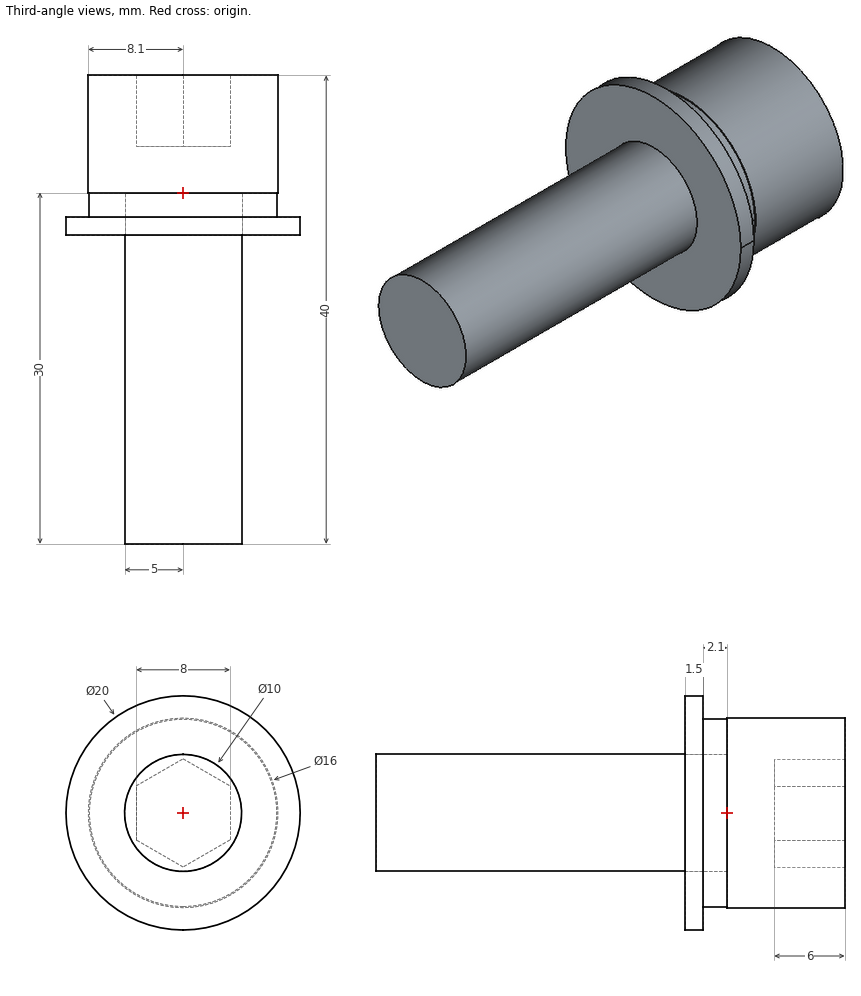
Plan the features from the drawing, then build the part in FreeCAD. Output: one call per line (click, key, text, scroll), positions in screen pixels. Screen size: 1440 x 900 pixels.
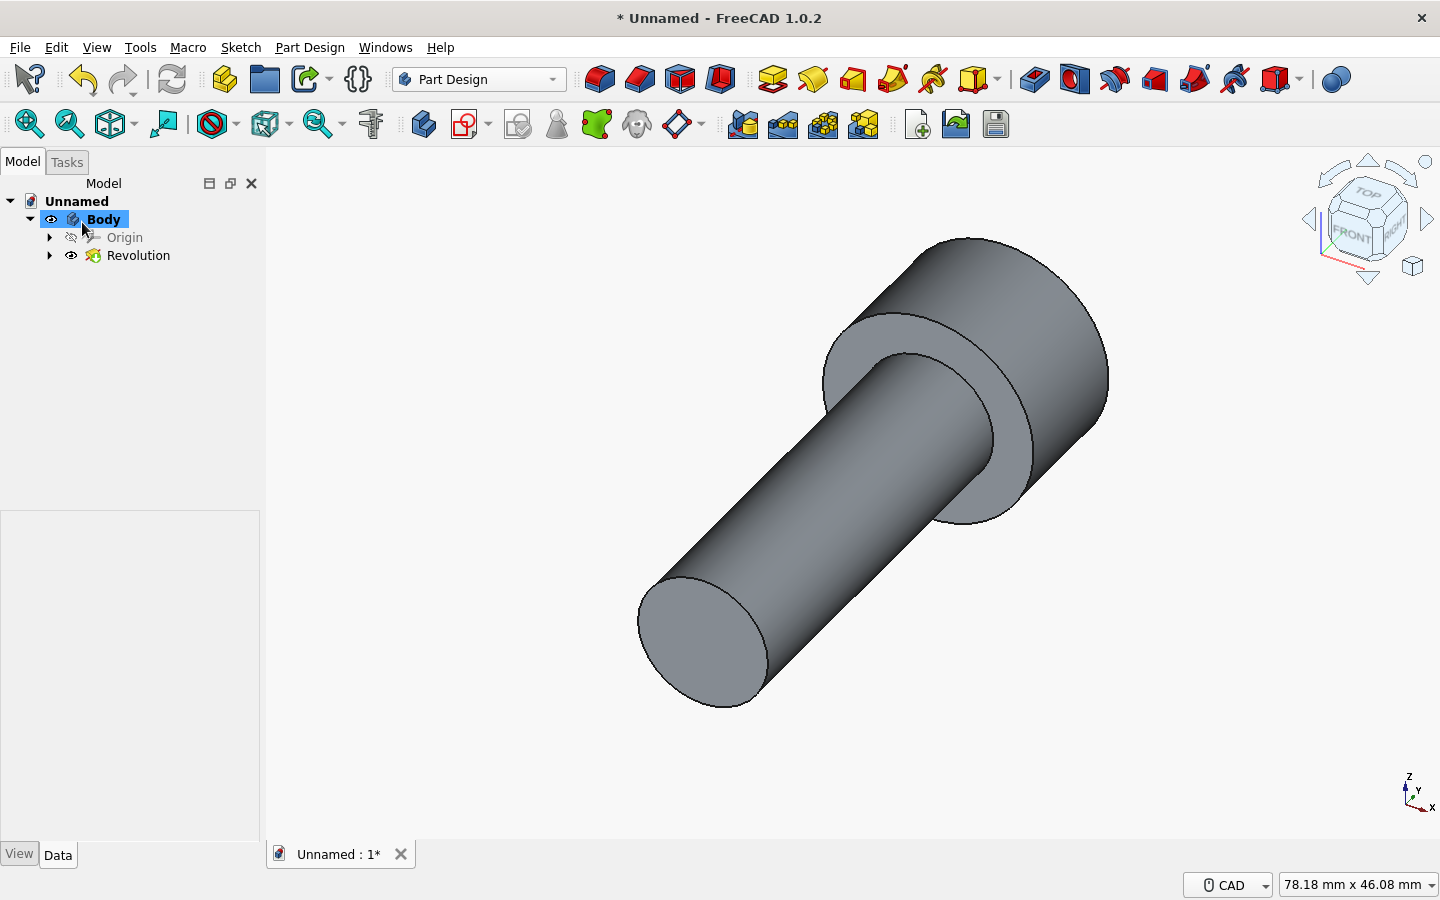
key(4)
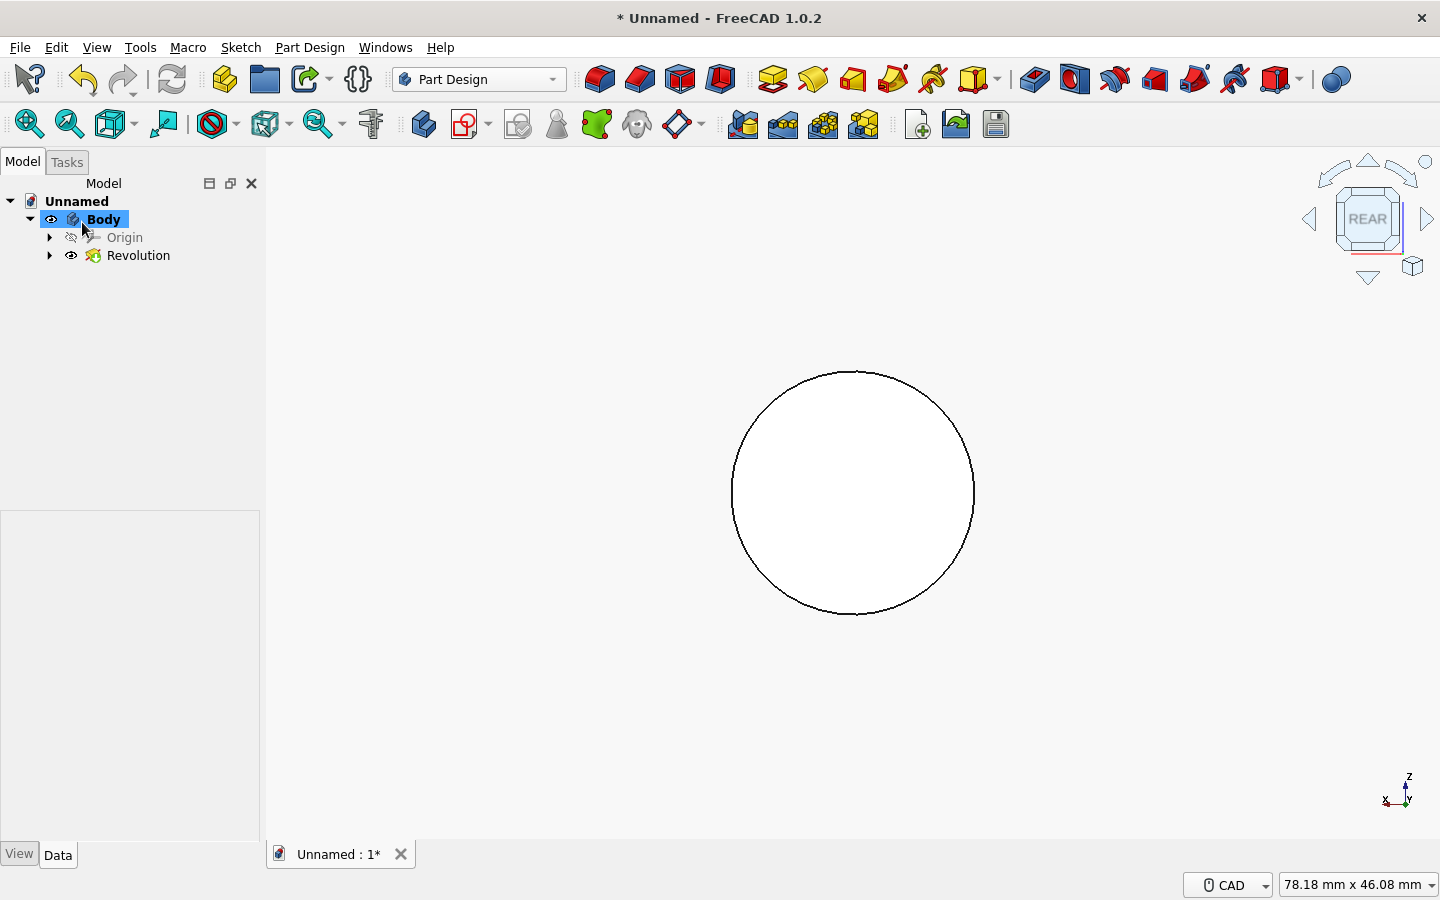
click(30, 124)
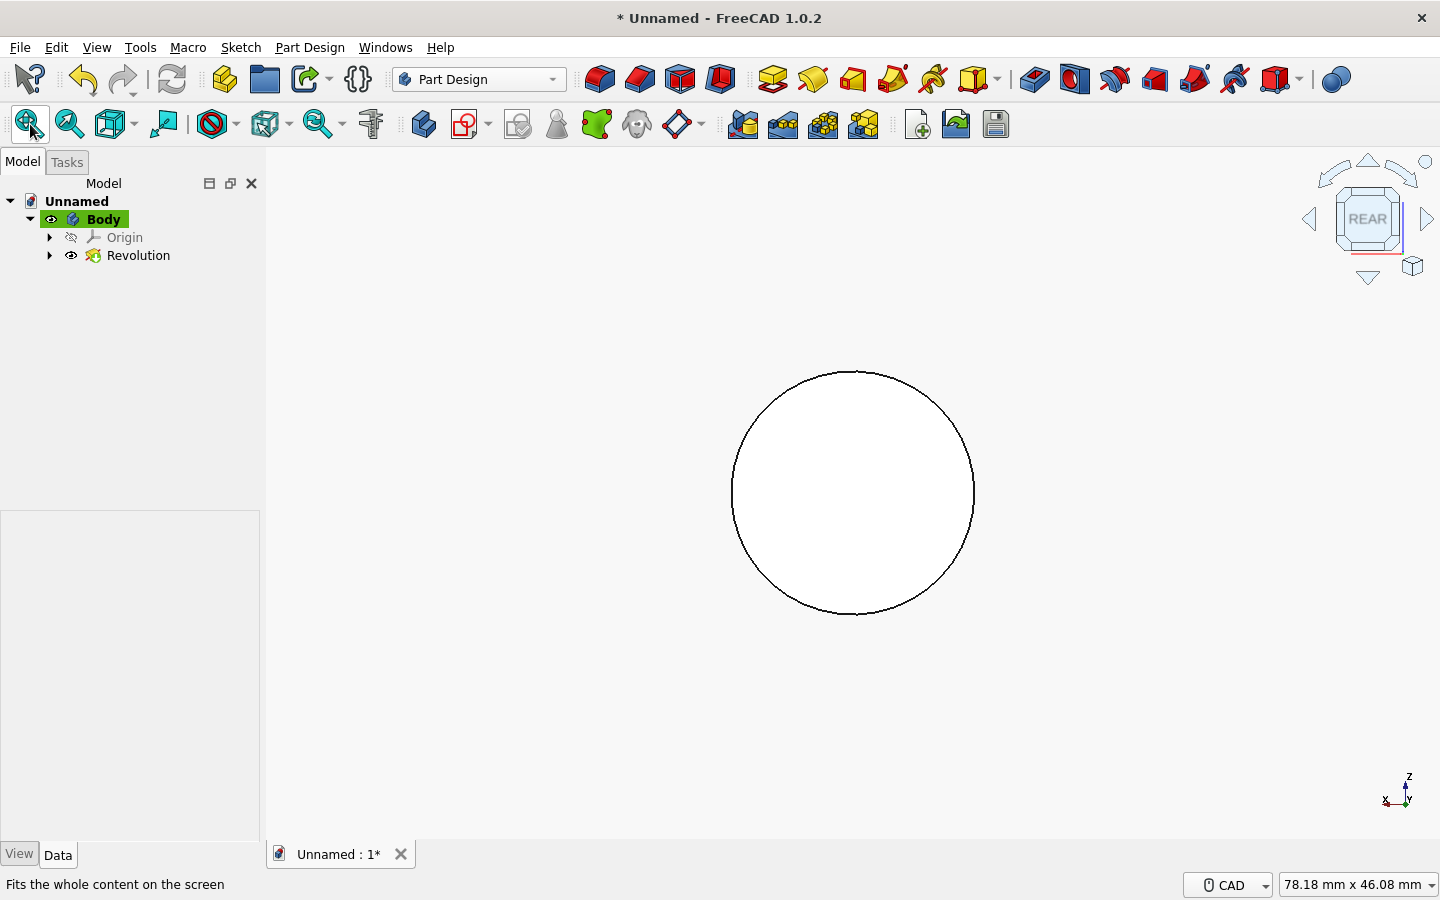
click(853, 492)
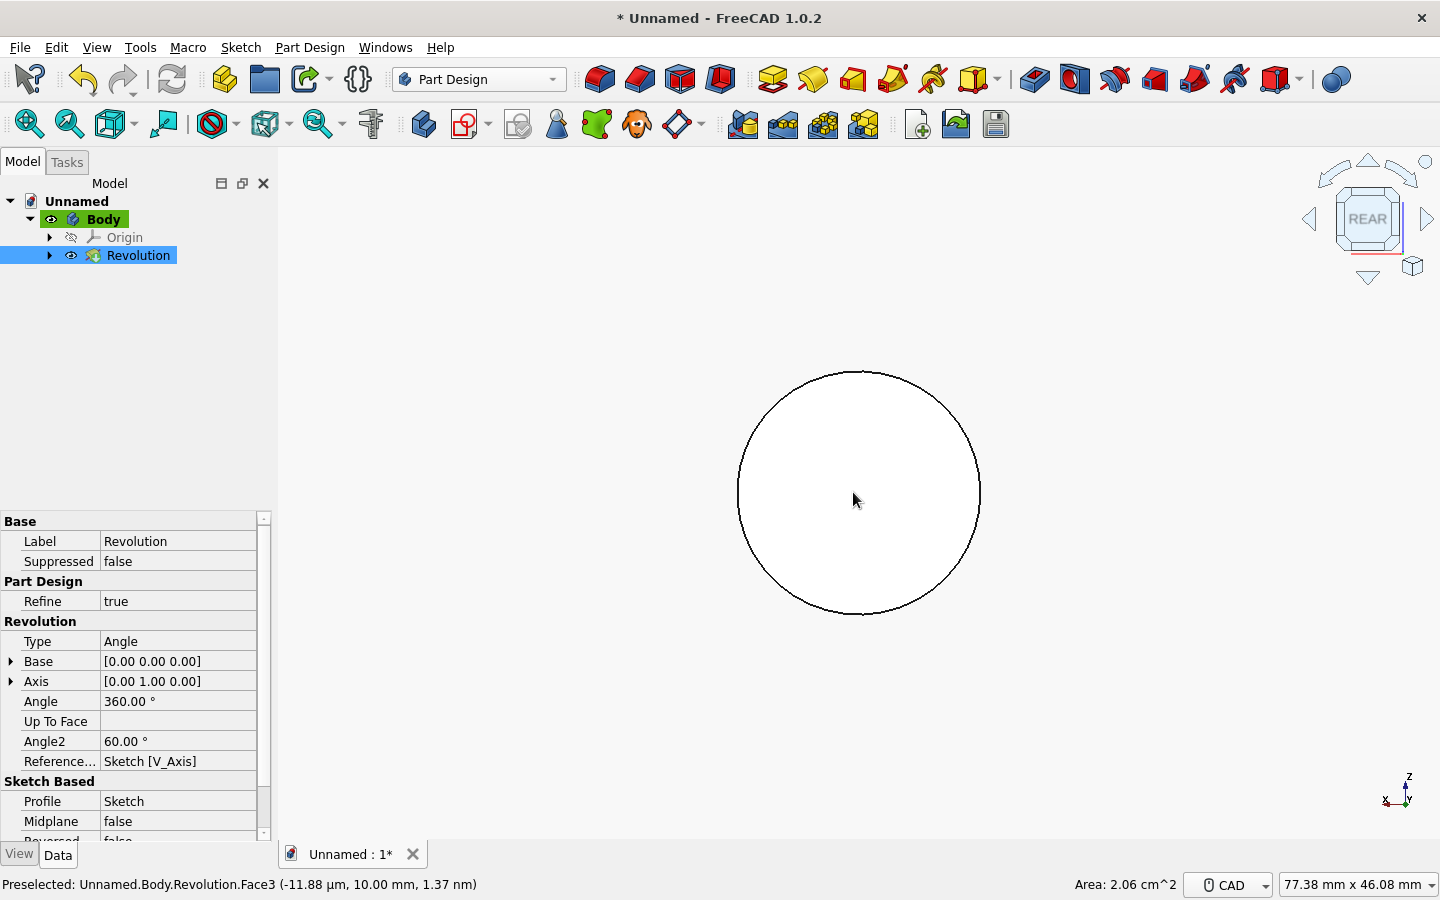
click(464, 124)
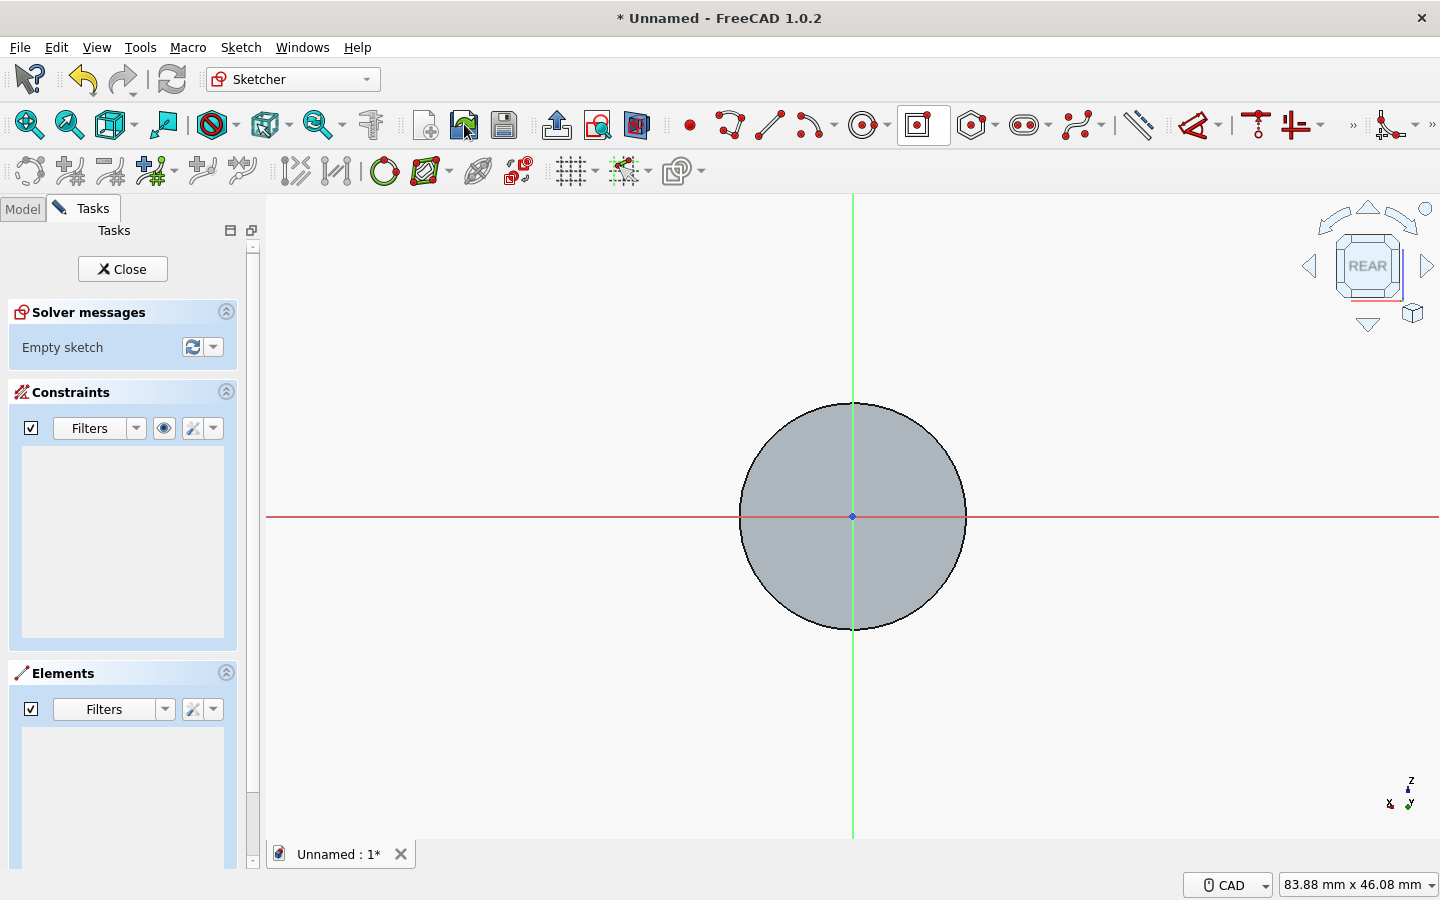
scroll(882, 516, up, 6)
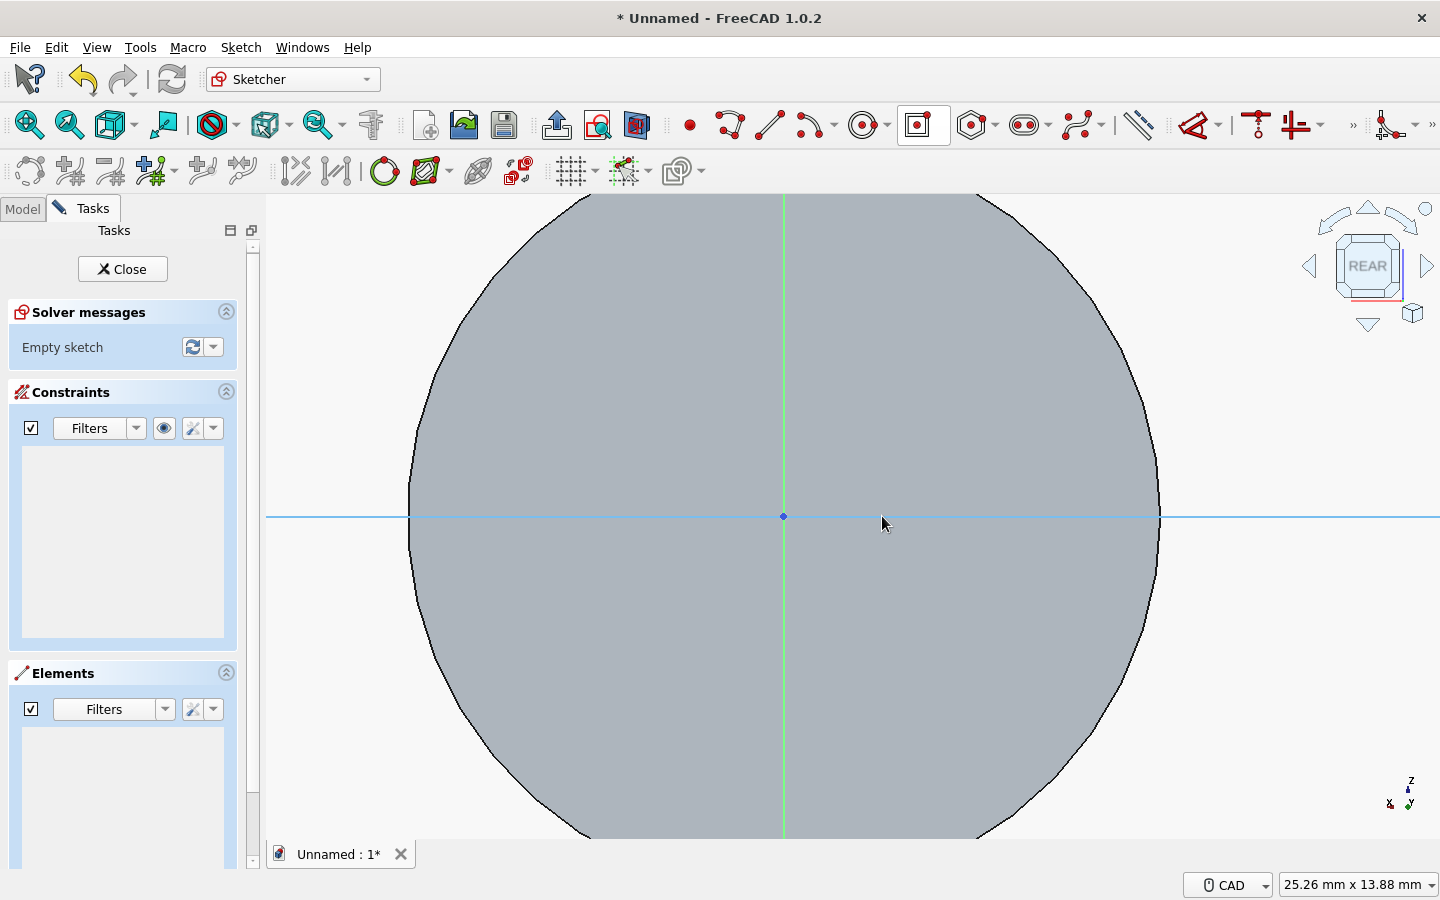
key(g)
key(p)
key(6)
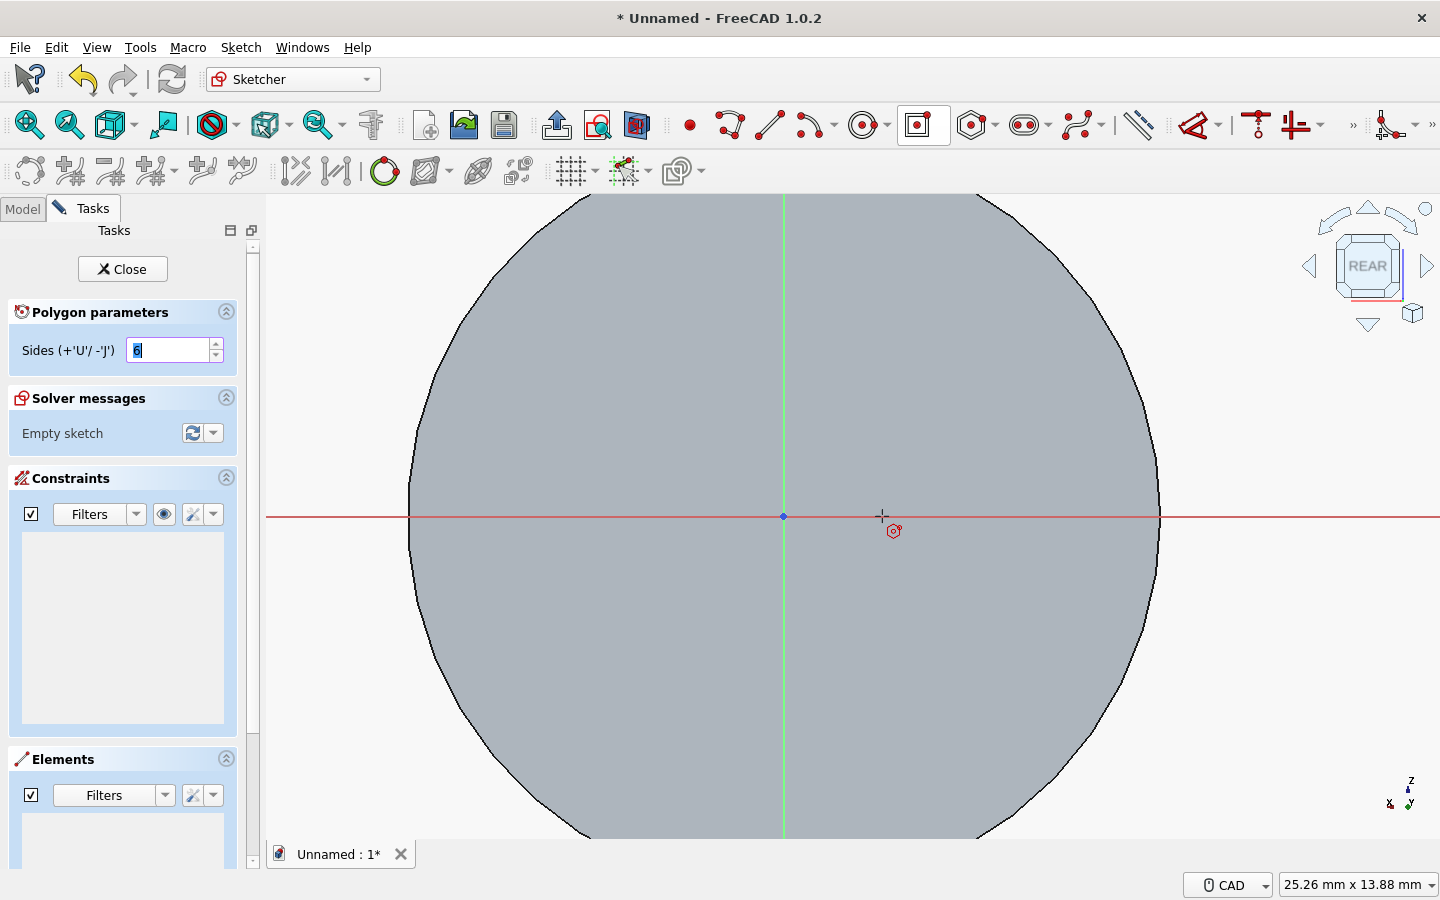
click(784, 516)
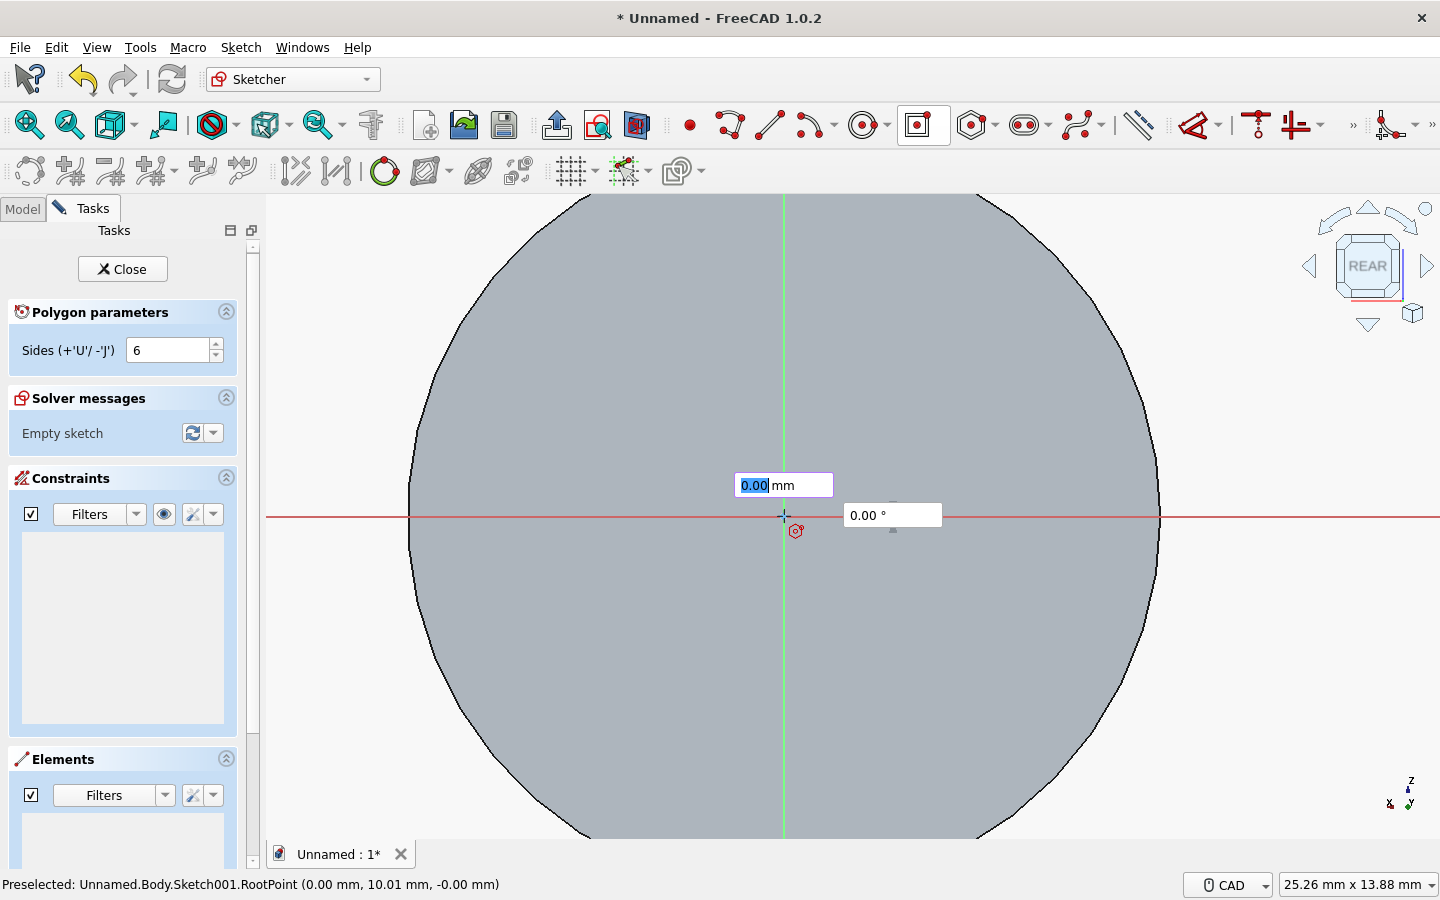
click(784, 731)
key(Escape)